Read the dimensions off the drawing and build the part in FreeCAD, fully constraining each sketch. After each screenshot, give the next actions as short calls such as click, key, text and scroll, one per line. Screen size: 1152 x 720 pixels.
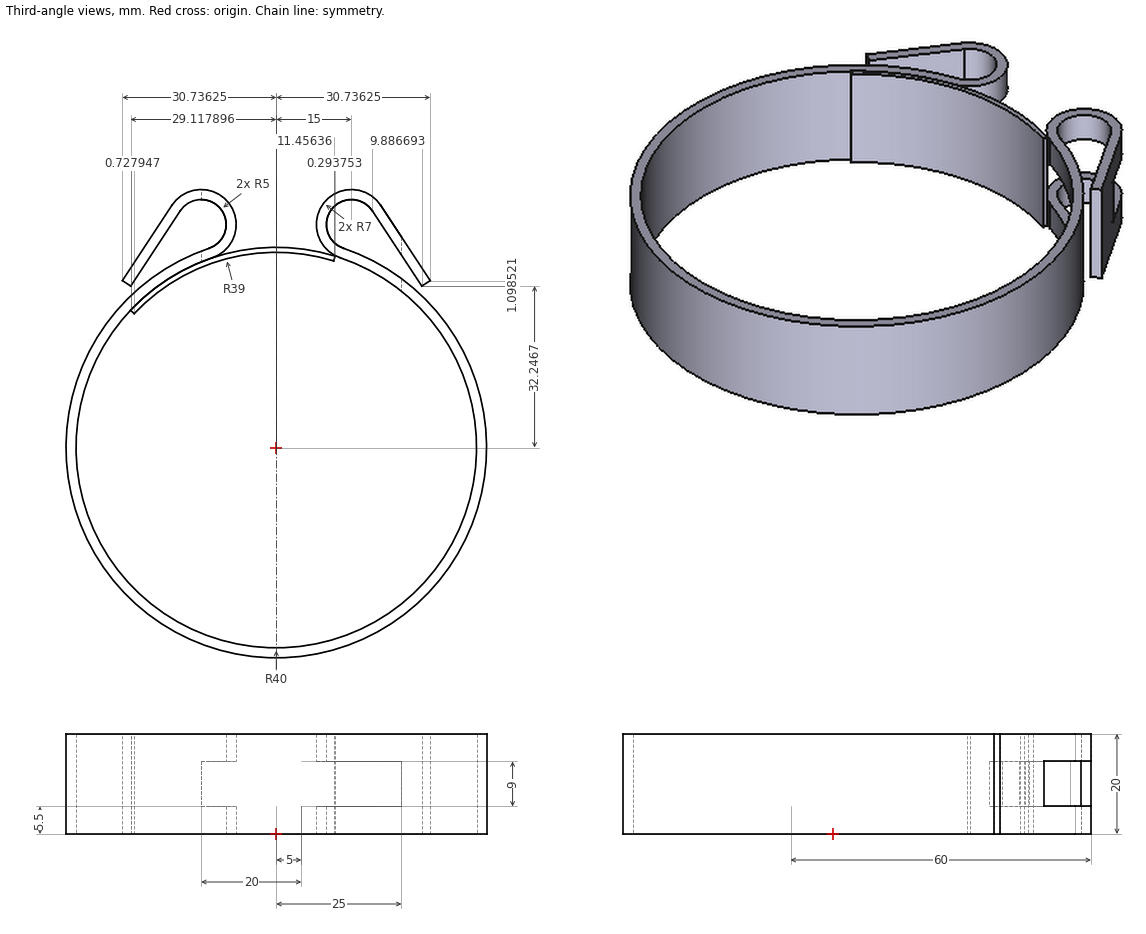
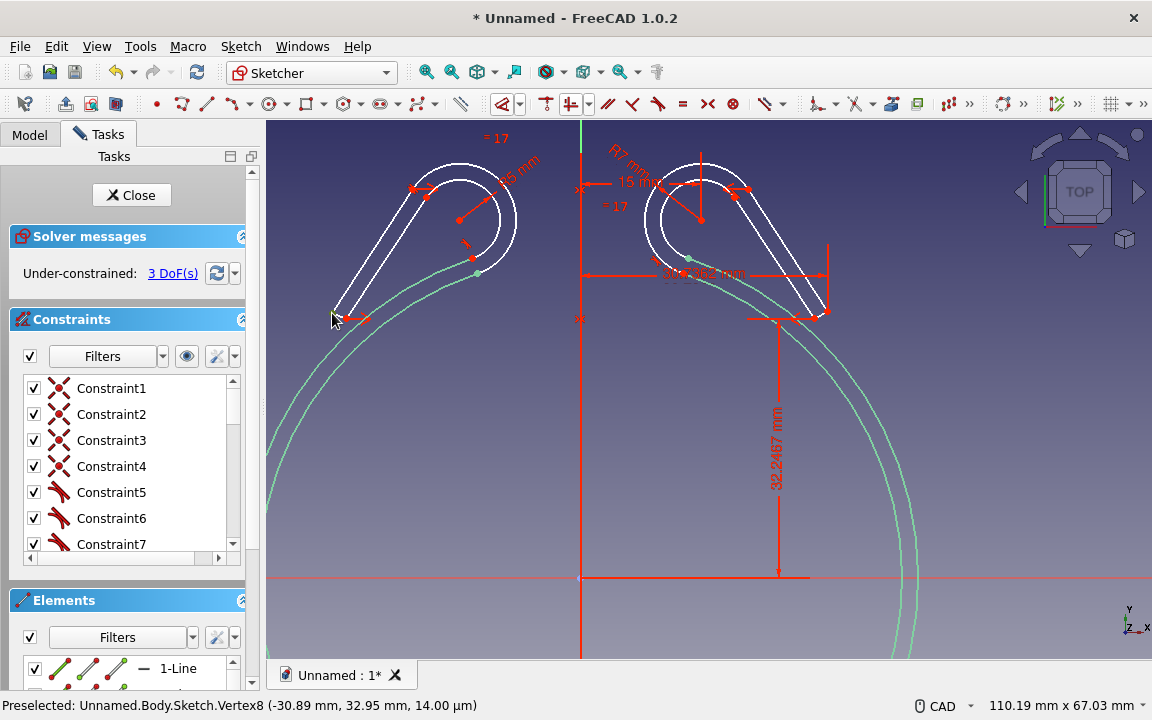
click(520, 104)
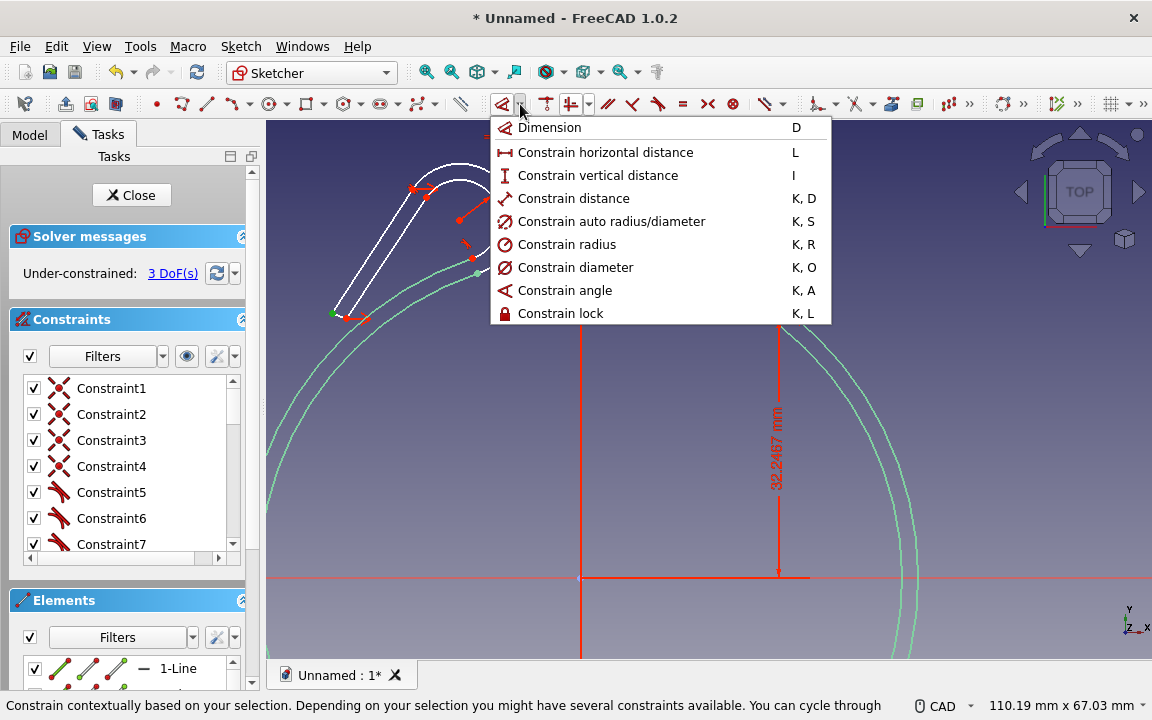
click(661, 152)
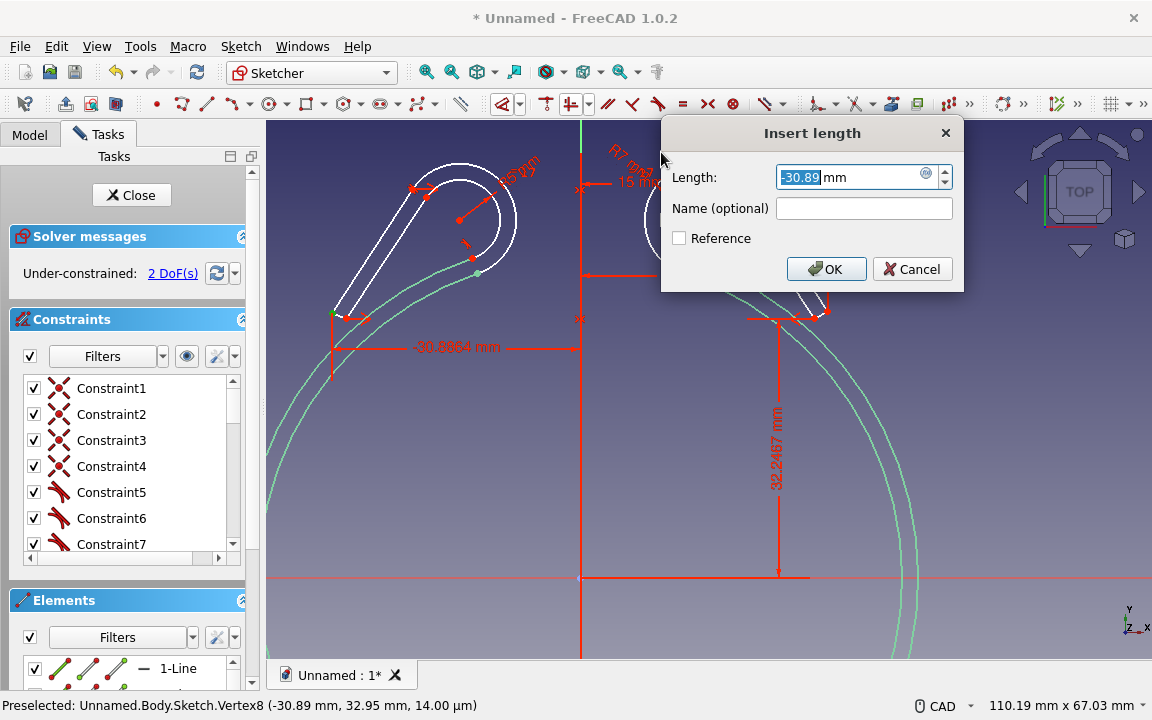
text(-30.73625)
key(Return)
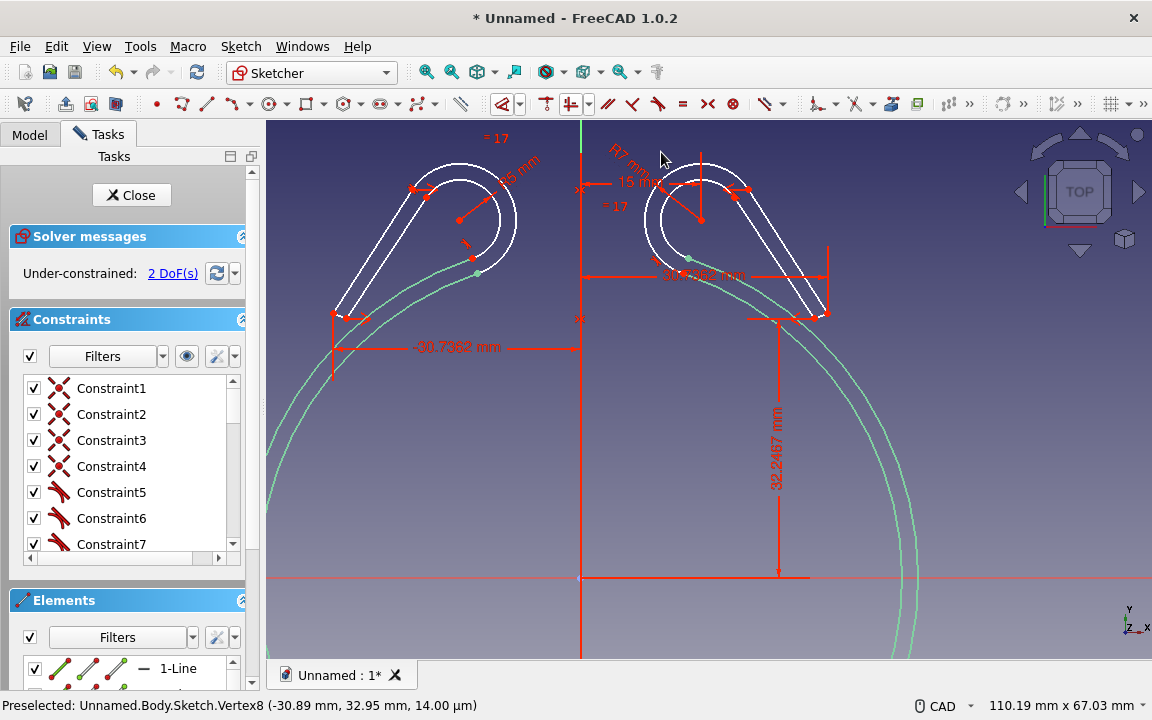
click(759, 234)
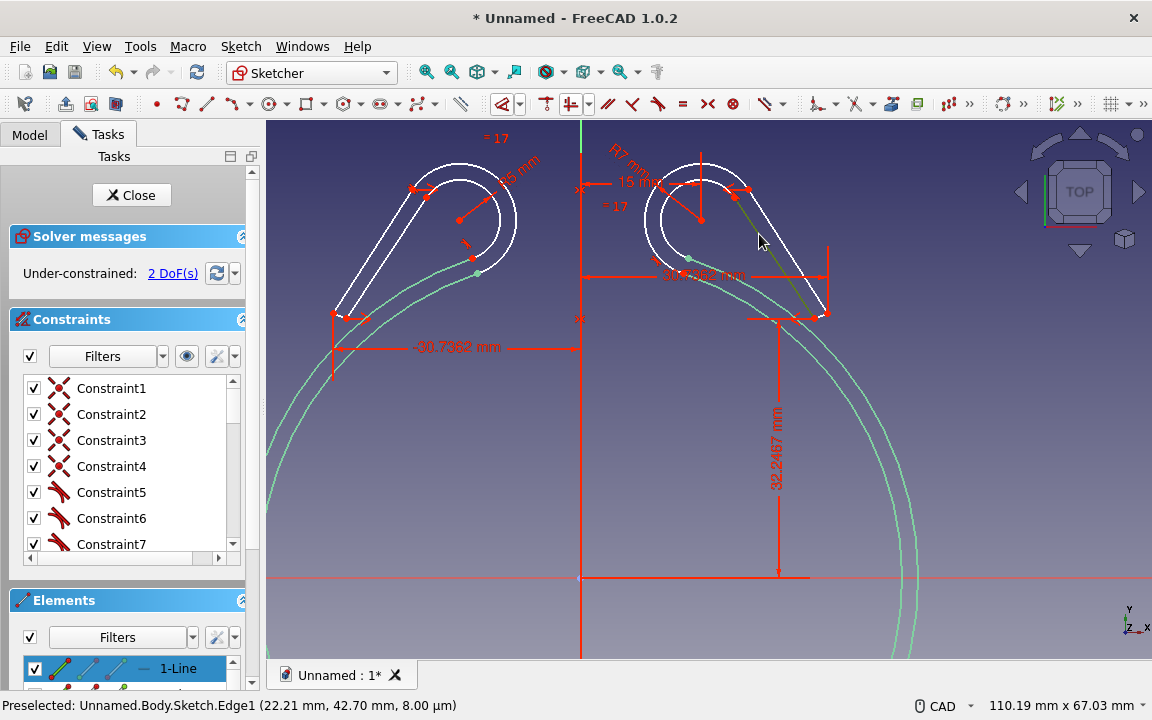
key(l)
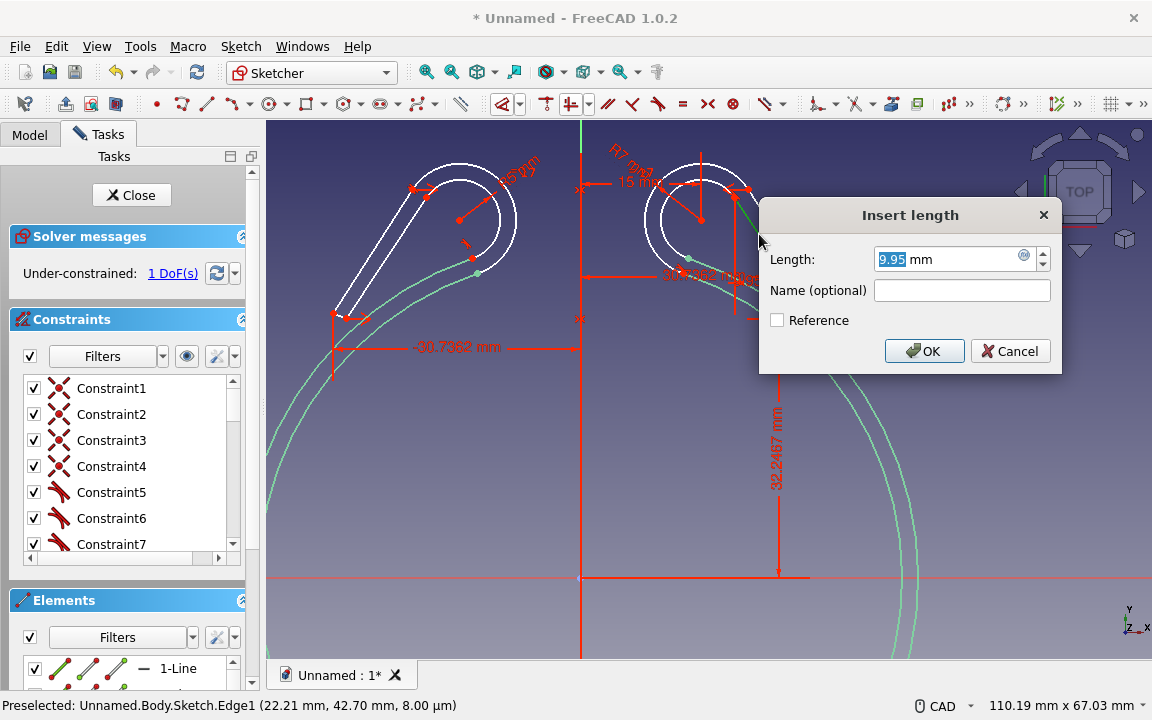
text(9.886693)
key(Return)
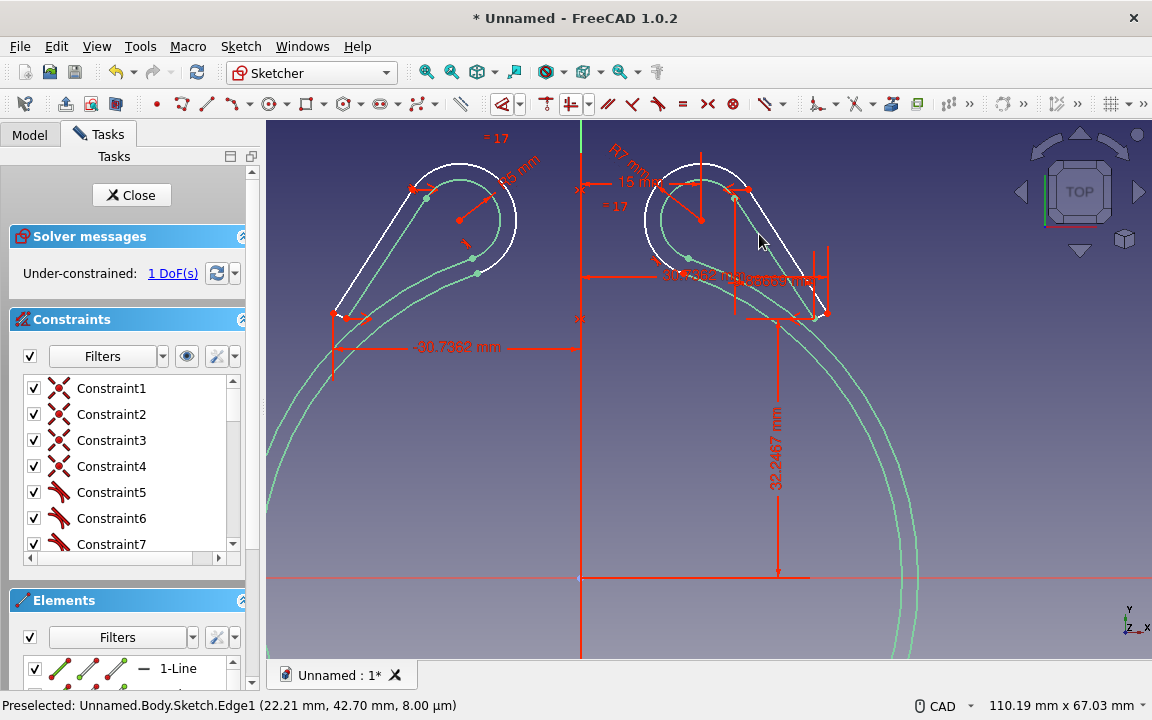
scroll(821, 316, up, 8)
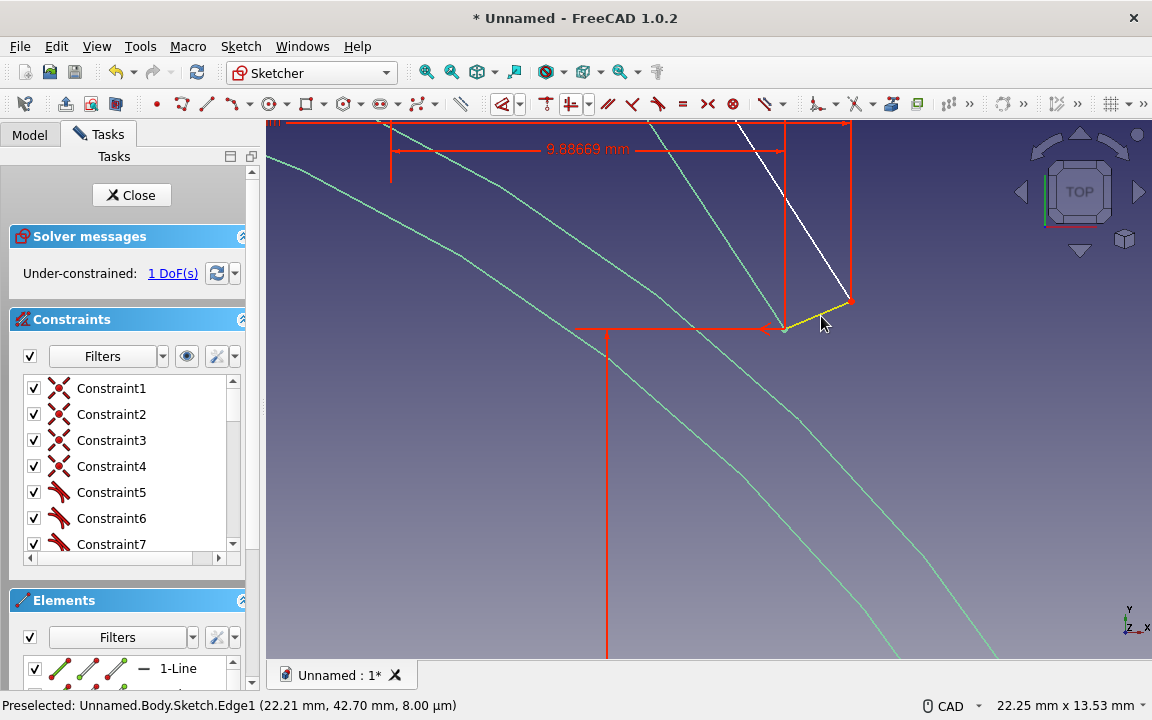
click(818, 315)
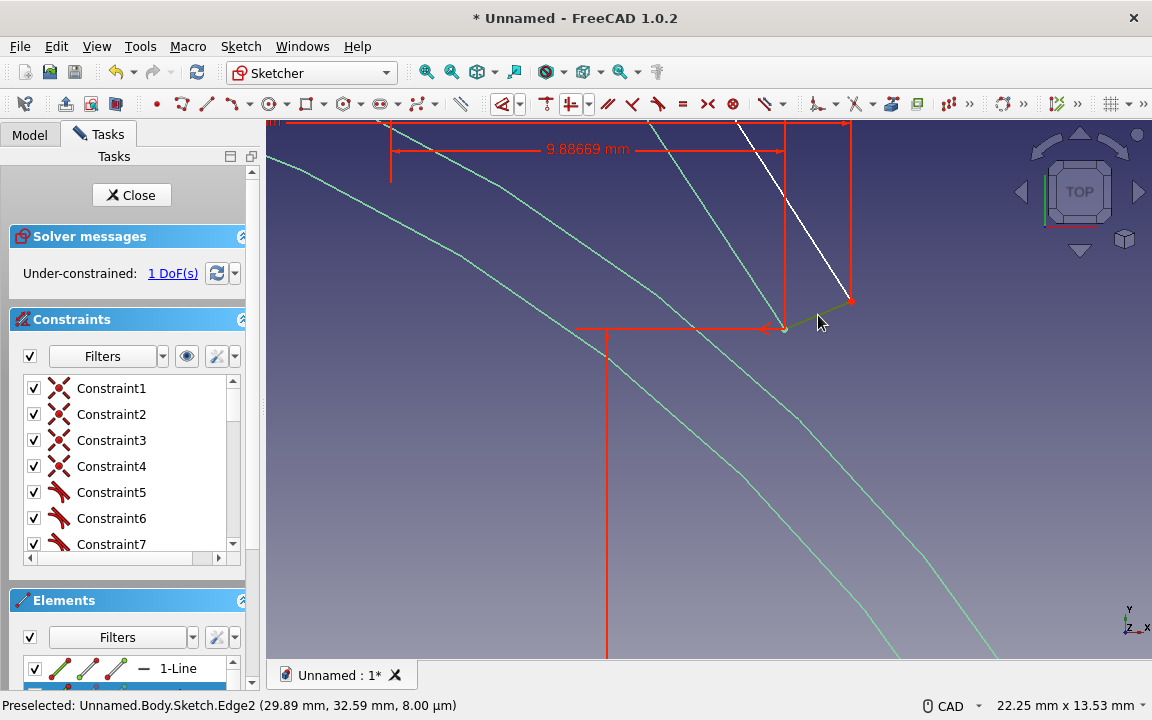
key(i)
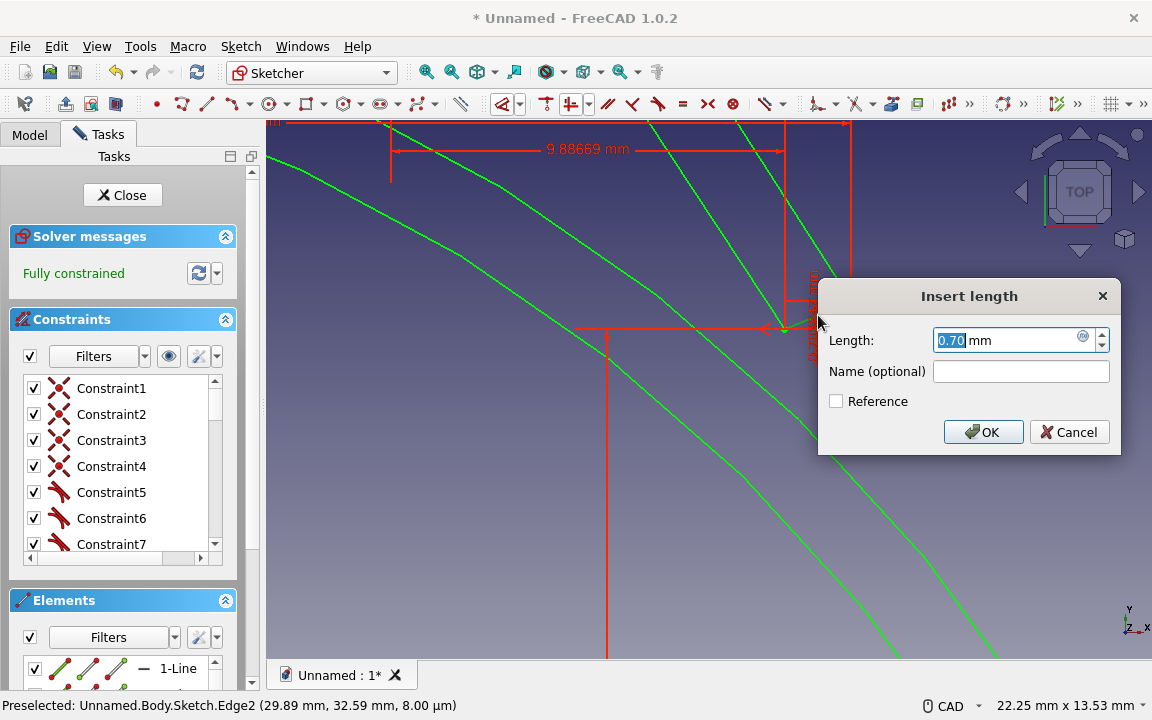
text(1.098521)
key(Return)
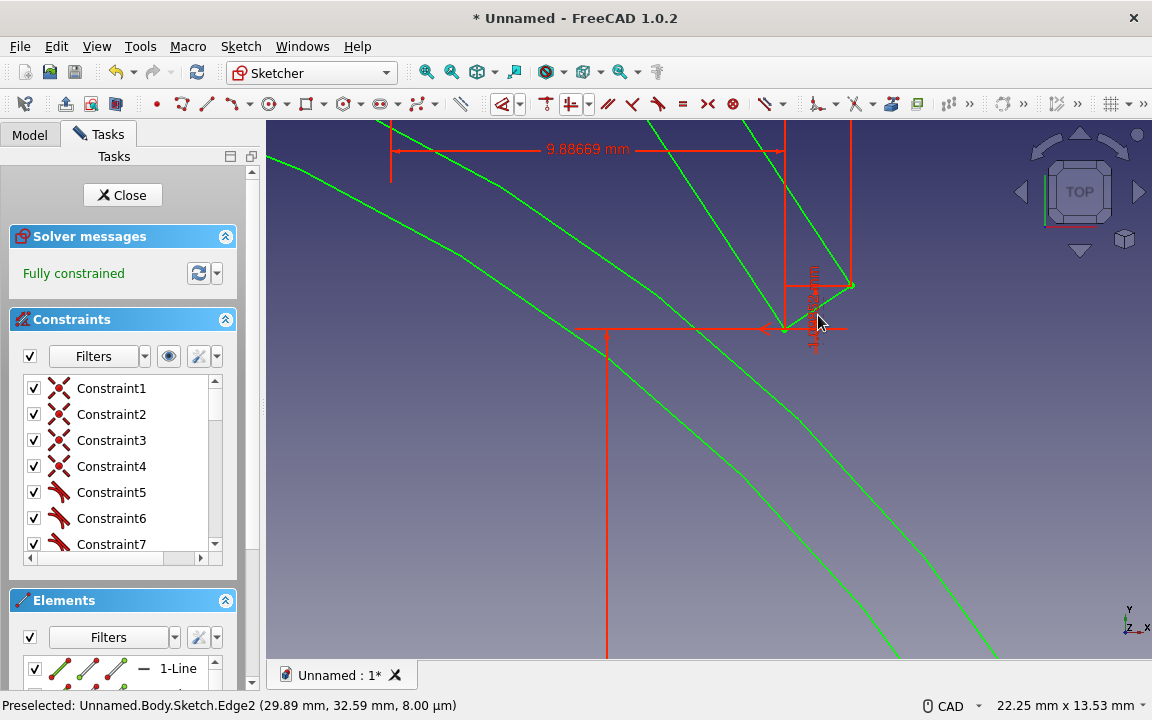
click(123, 195)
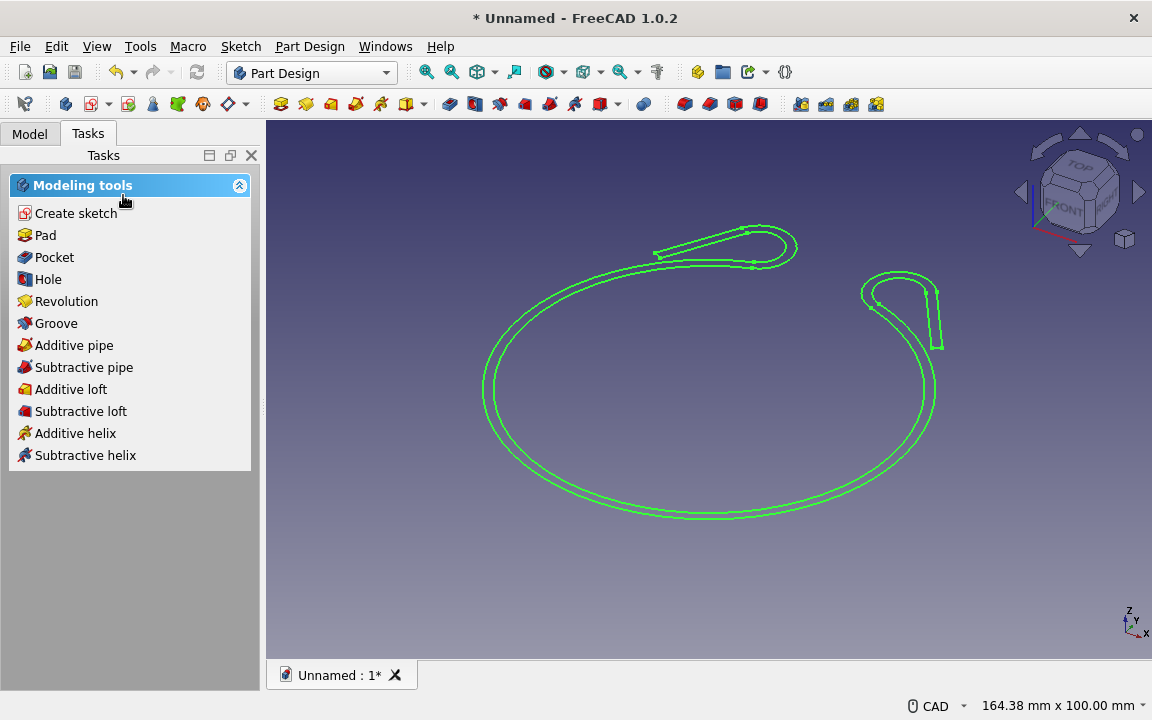
click(281, 104)